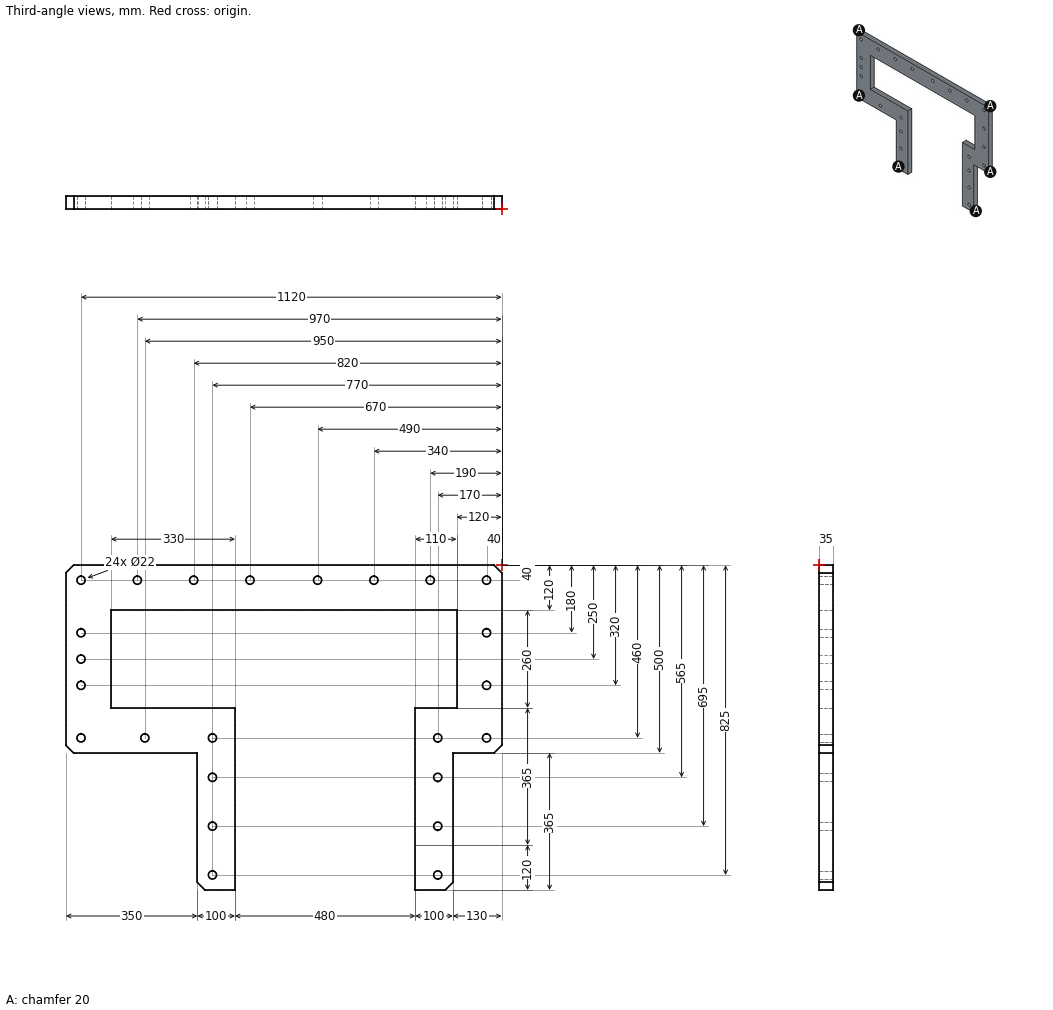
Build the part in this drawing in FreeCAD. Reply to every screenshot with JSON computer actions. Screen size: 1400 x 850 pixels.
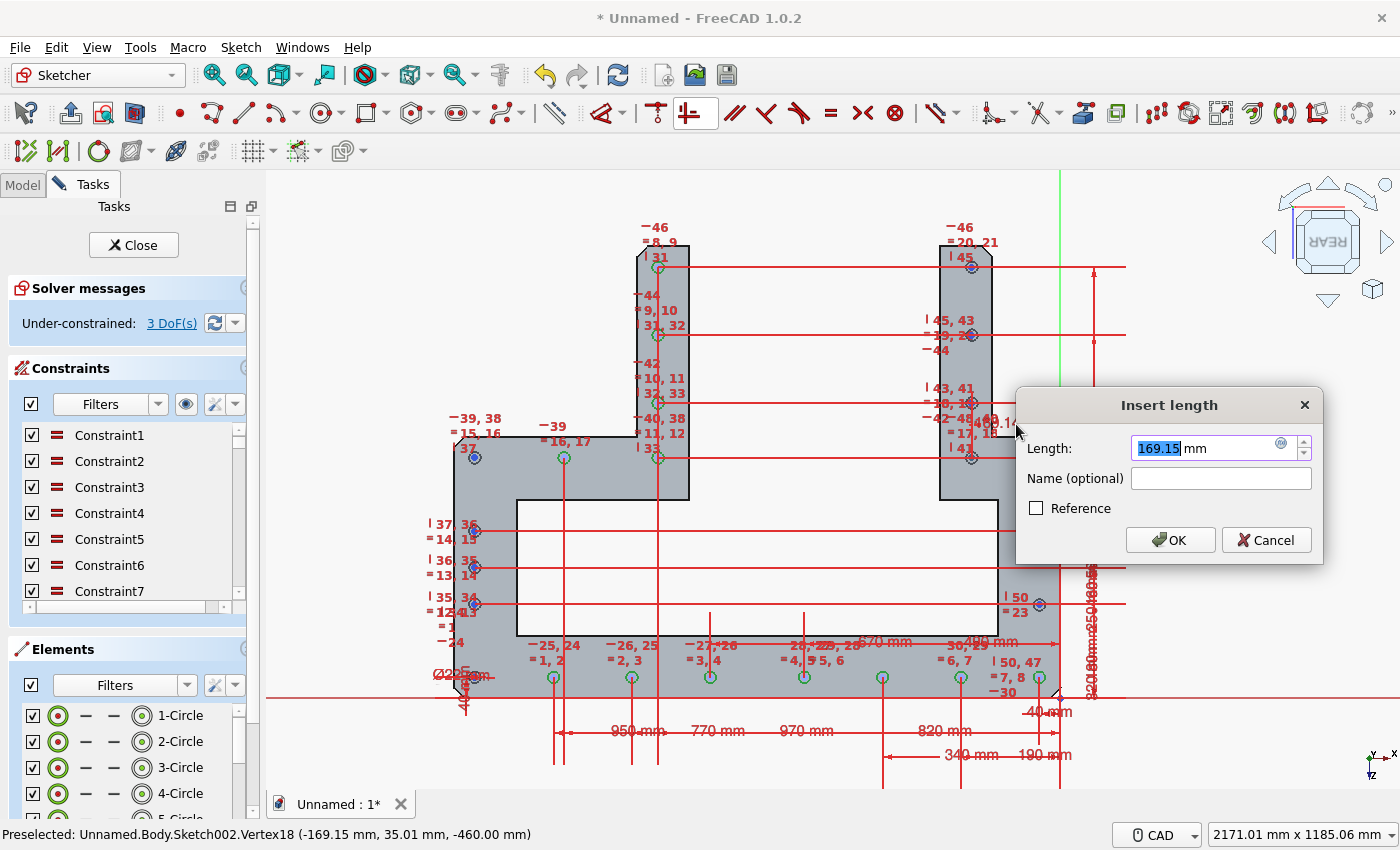
{"action": "type", "text": "170"}
{"action": "key", "text": "Return"}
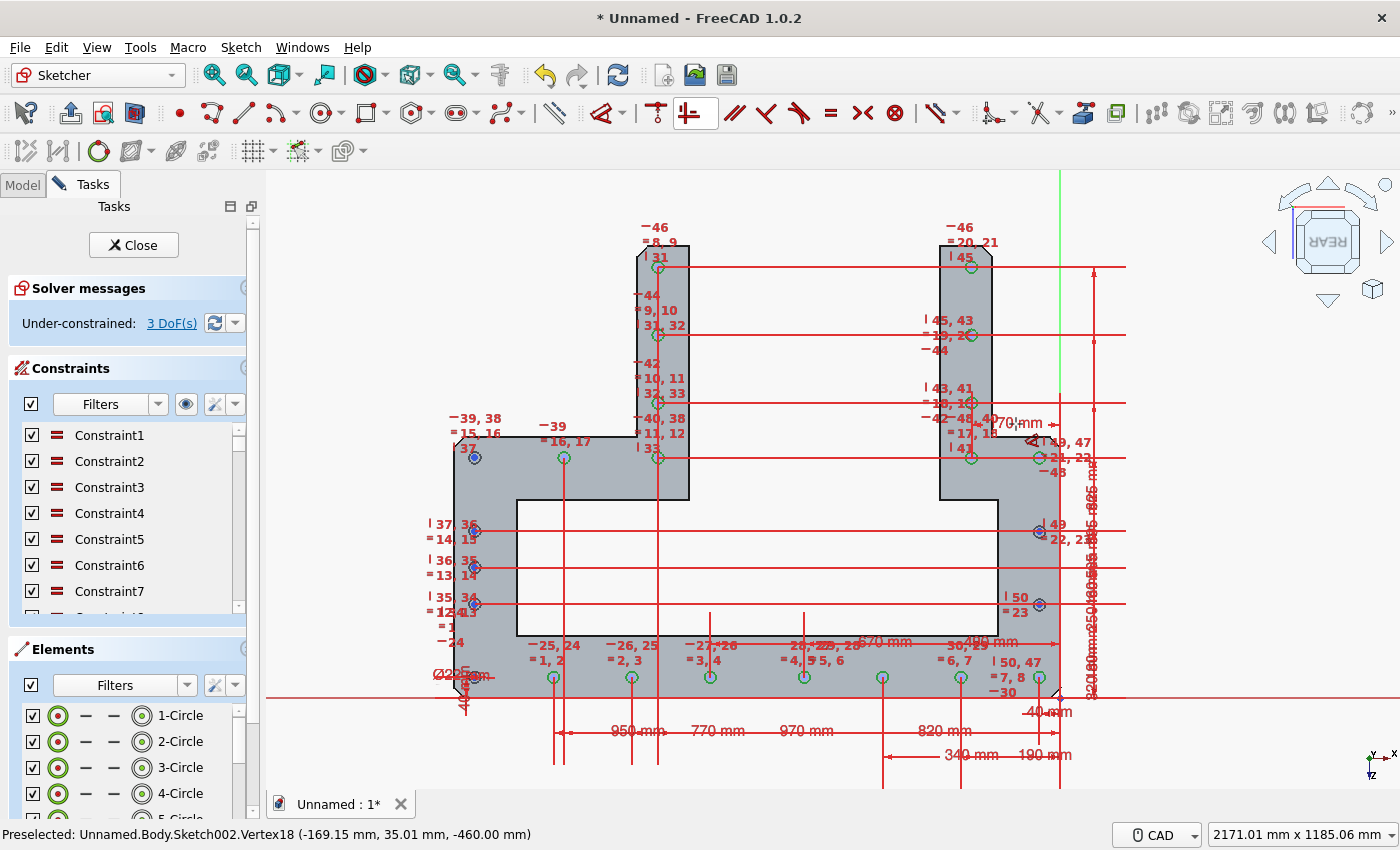
{"action": "left_click", "coordinate": [1039, 532]}
{"action": "left_click", "coordinate": [1005, 615]}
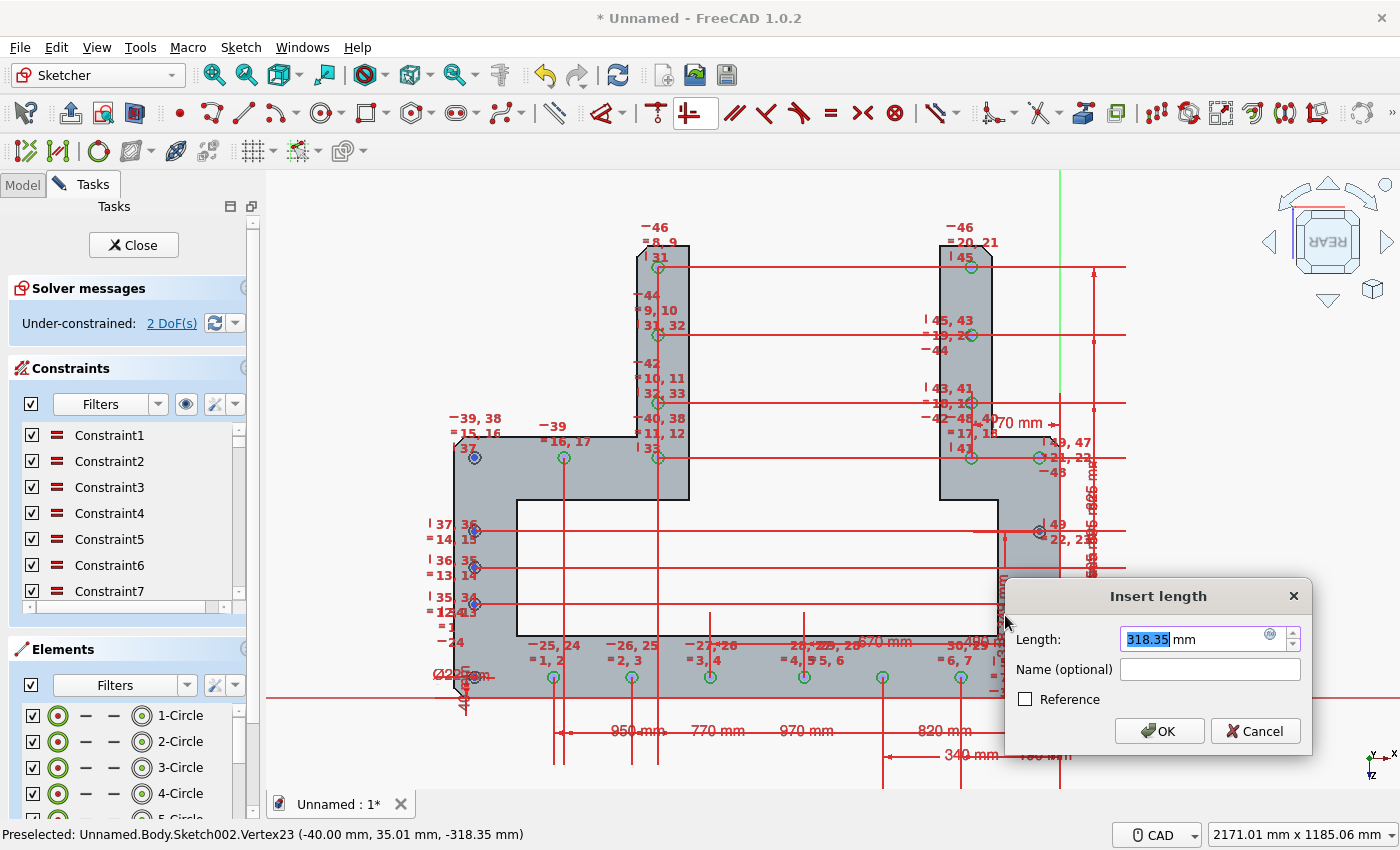
{"action": "type", "text": "320"}
{"action": "key", "text": "Return"}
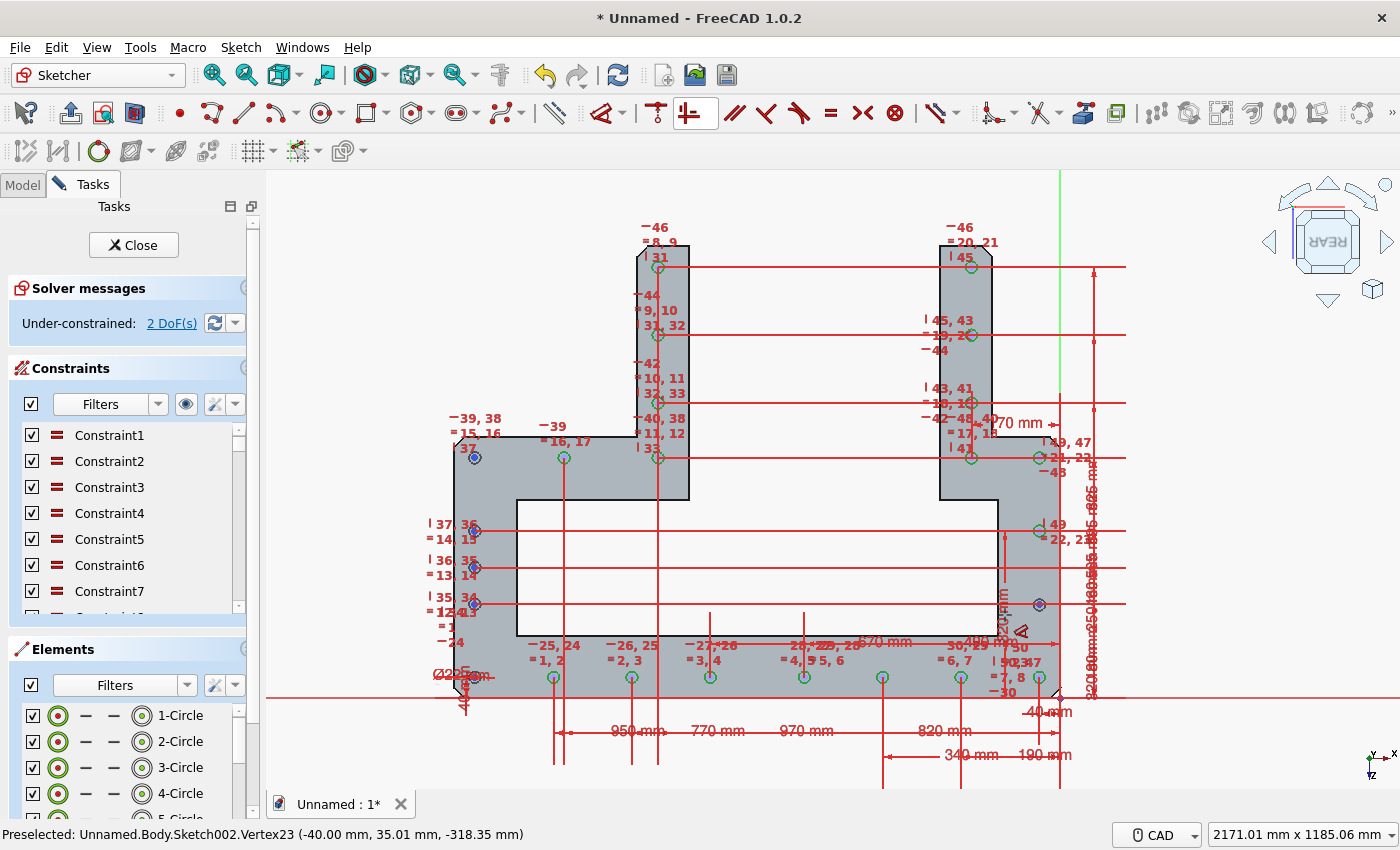
{"action": "left_click", "coordinate": [1039, 605]}
{"action": "left_click", "coordinate": [1094, 630]}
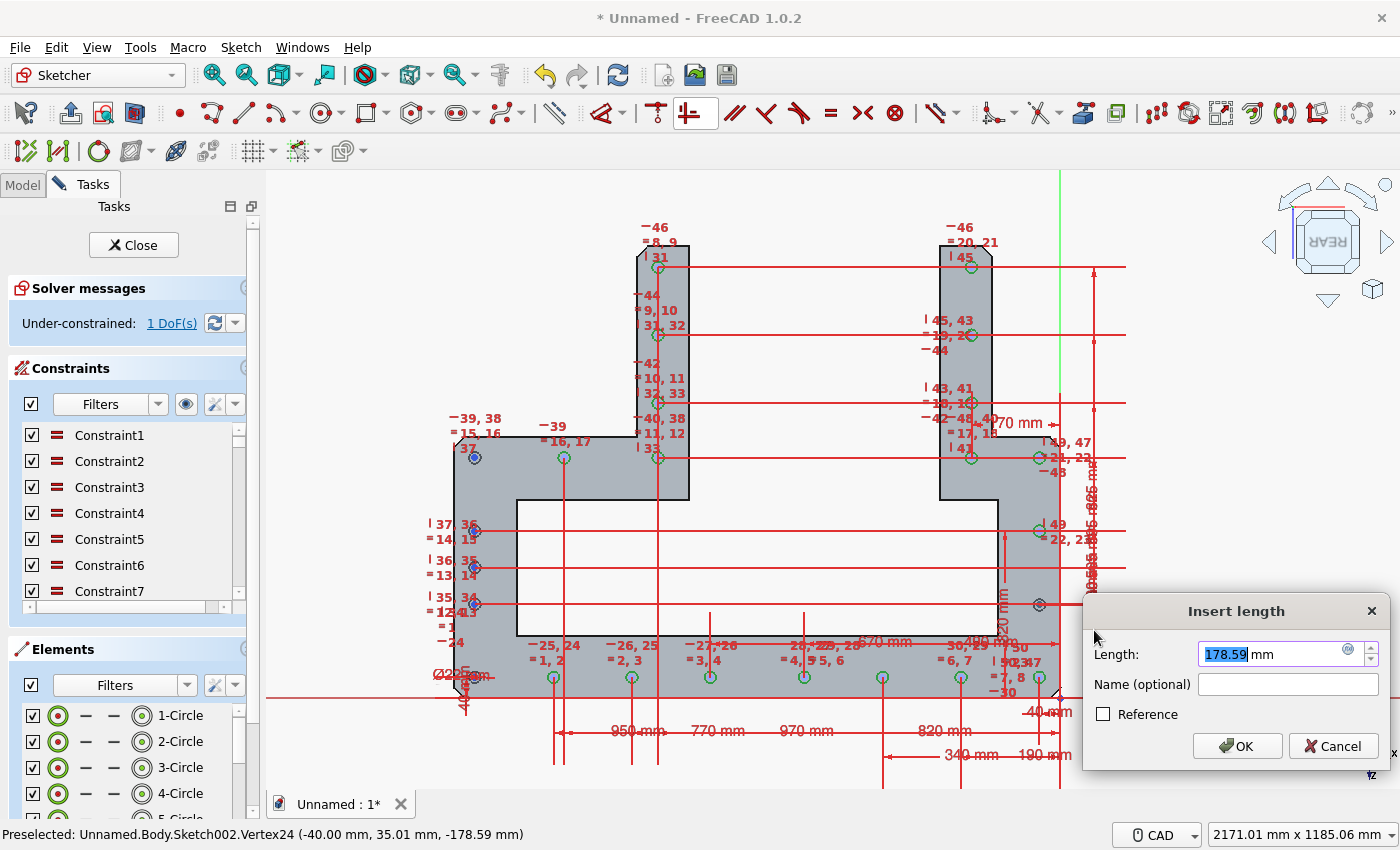
{"action": "type", "text": "180"}
{"action": "key", "text": "Return"}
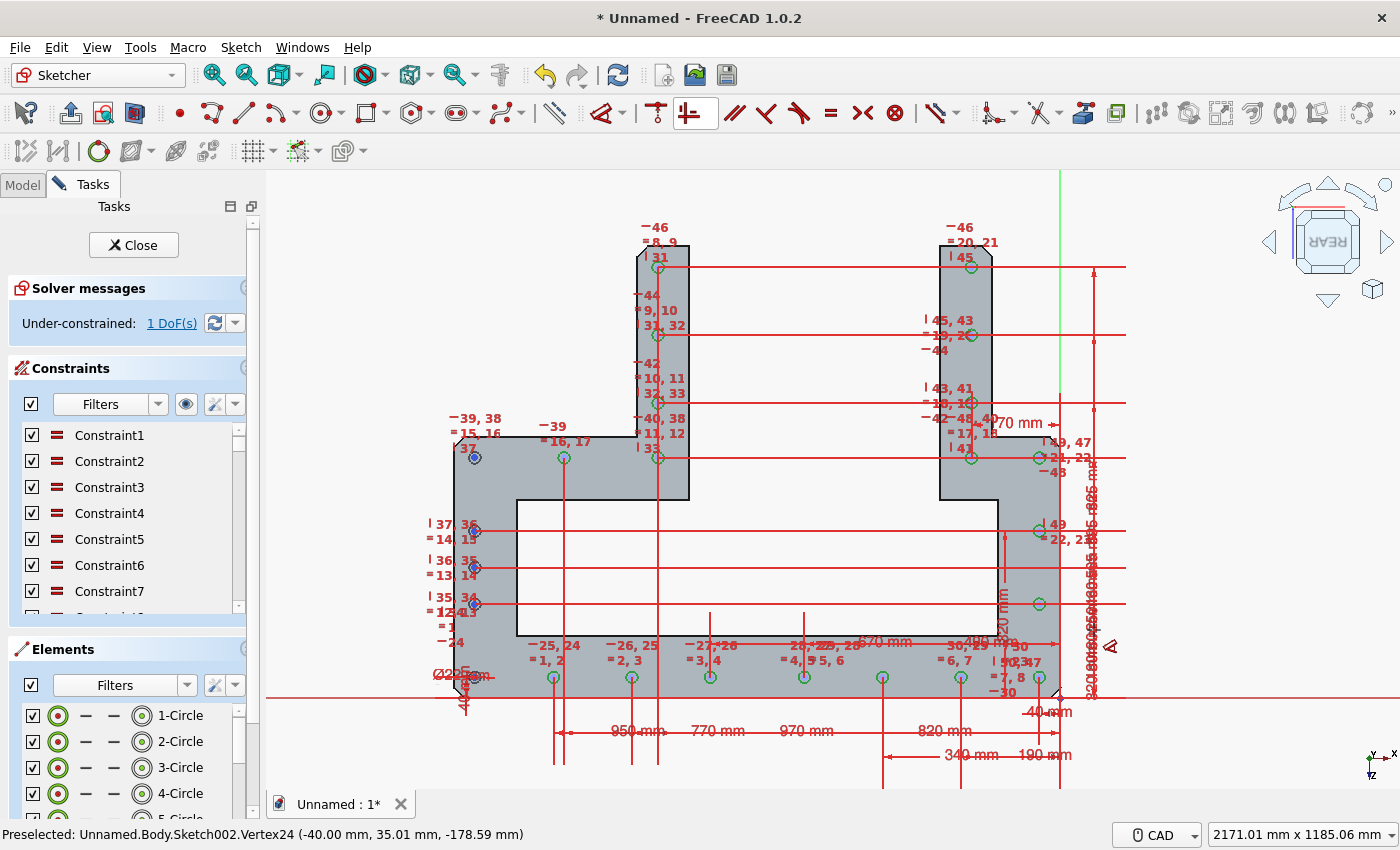
{"action": "left_click", "coordinate": [475, 677]}
{"action": "left_click", "coordinate": [563, 732]}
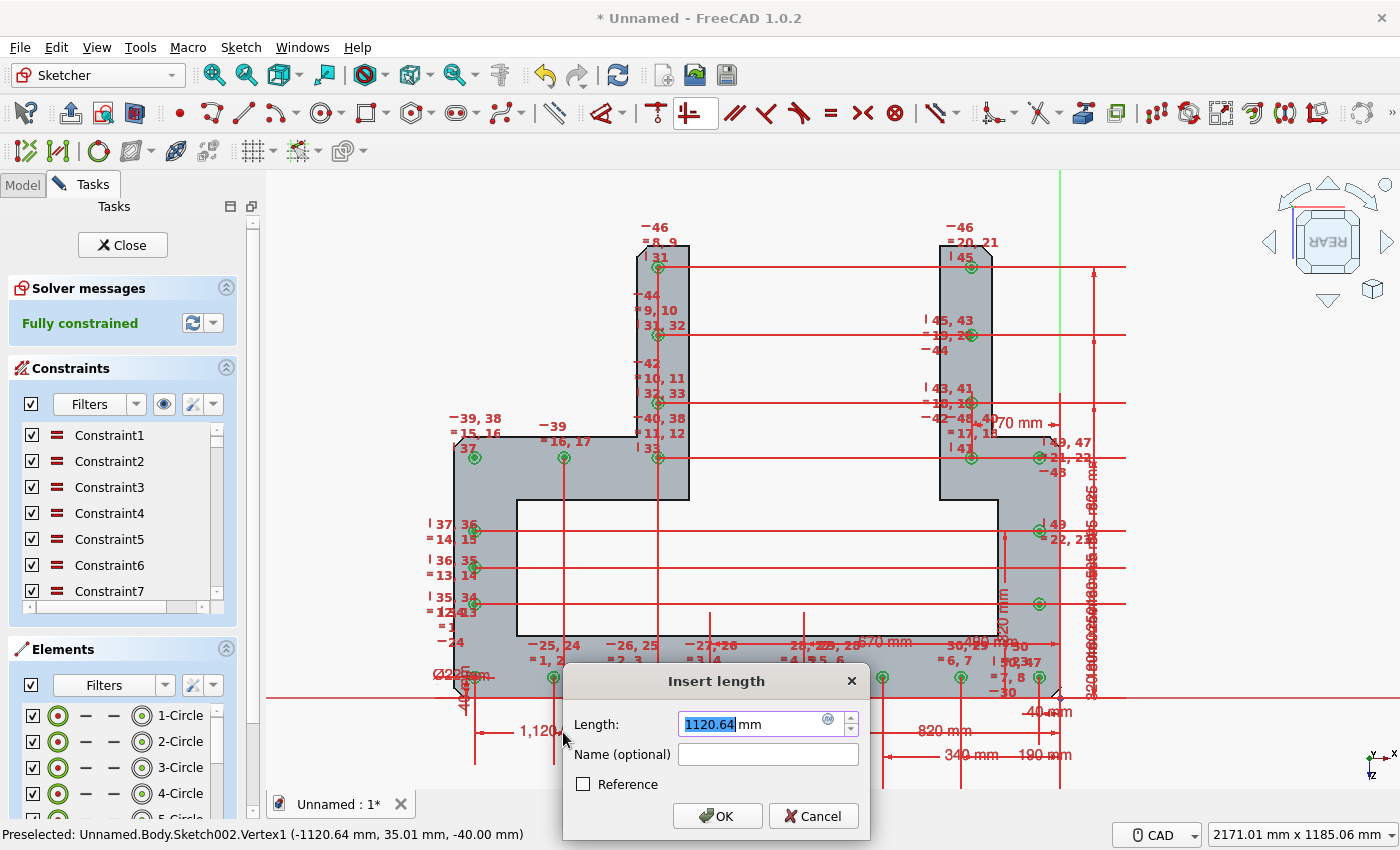
{"action": "type", "text": "1120"}
{"action": "key", "text": "Return"}
{"action": "key", "text": "Escape"}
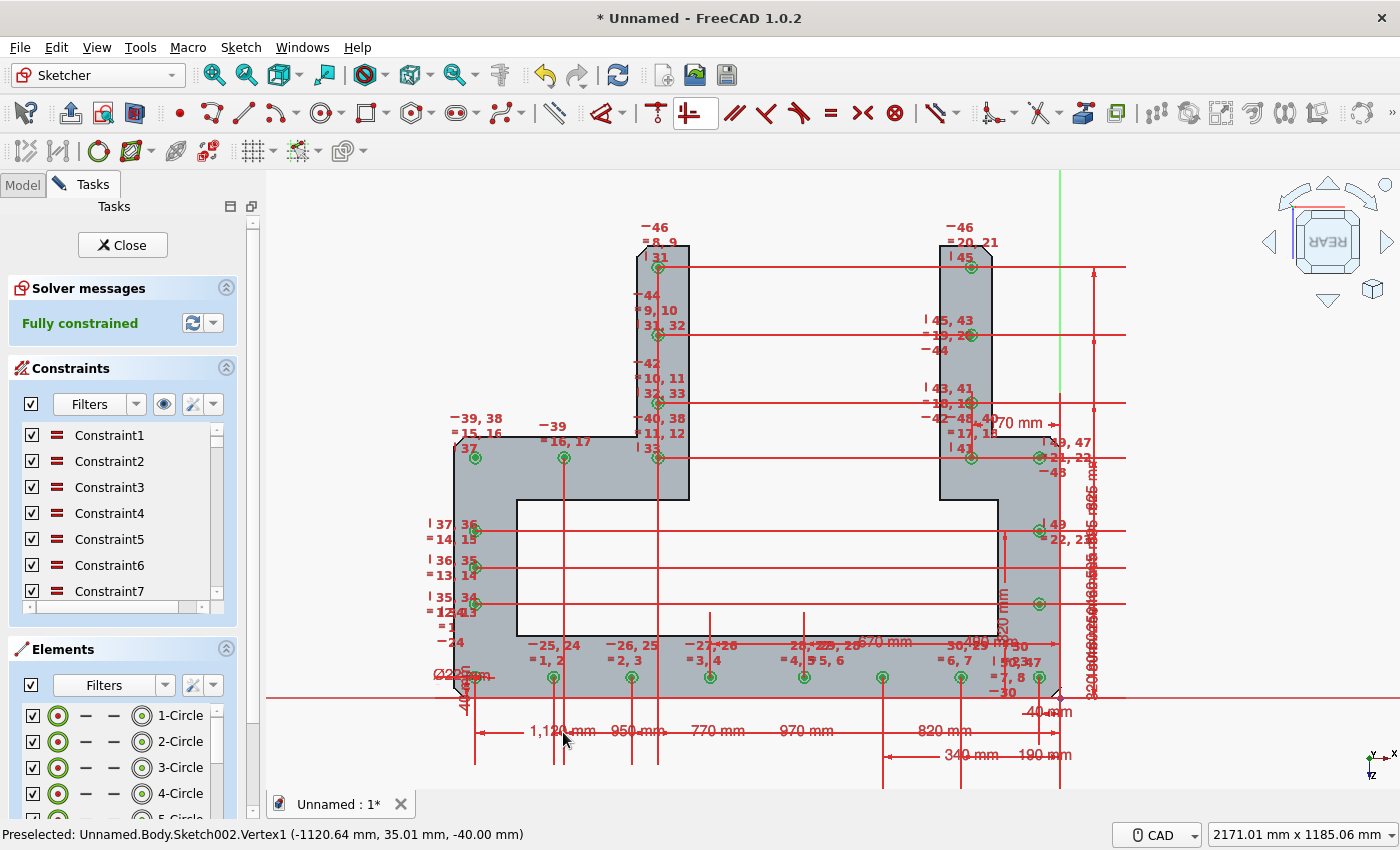
{"action": "left_click", "coordinate": [123, 245]}